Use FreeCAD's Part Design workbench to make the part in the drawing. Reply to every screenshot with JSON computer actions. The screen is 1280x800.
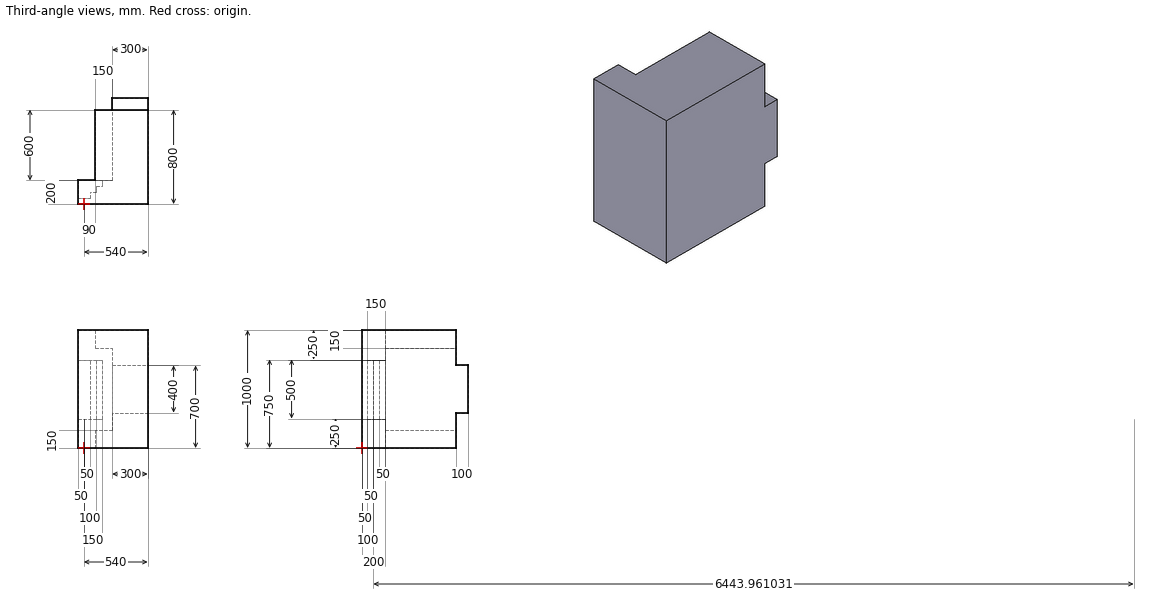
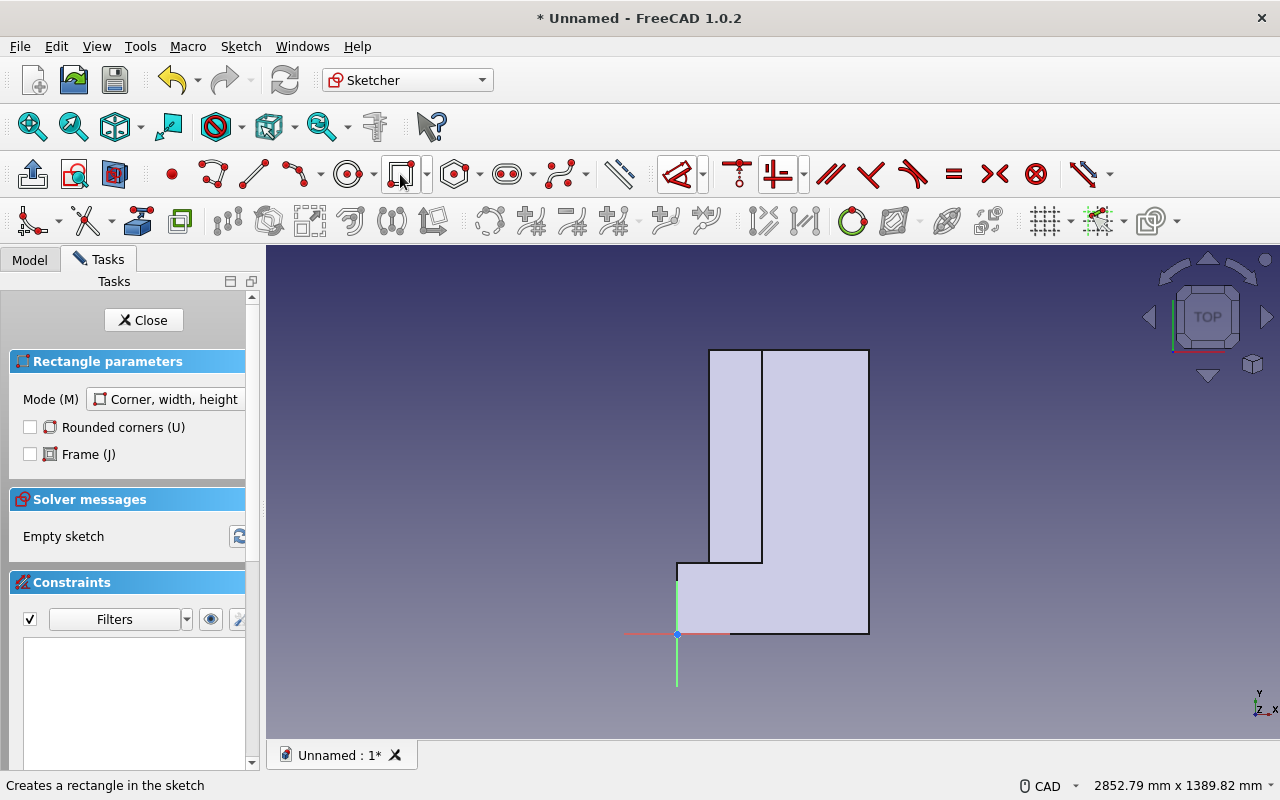
{"action": "left_click", "coordinate": [709, 350]}
{"action": "left_click", "coordinate": [762, 563]}
{"action": "key", "text": "Escape"}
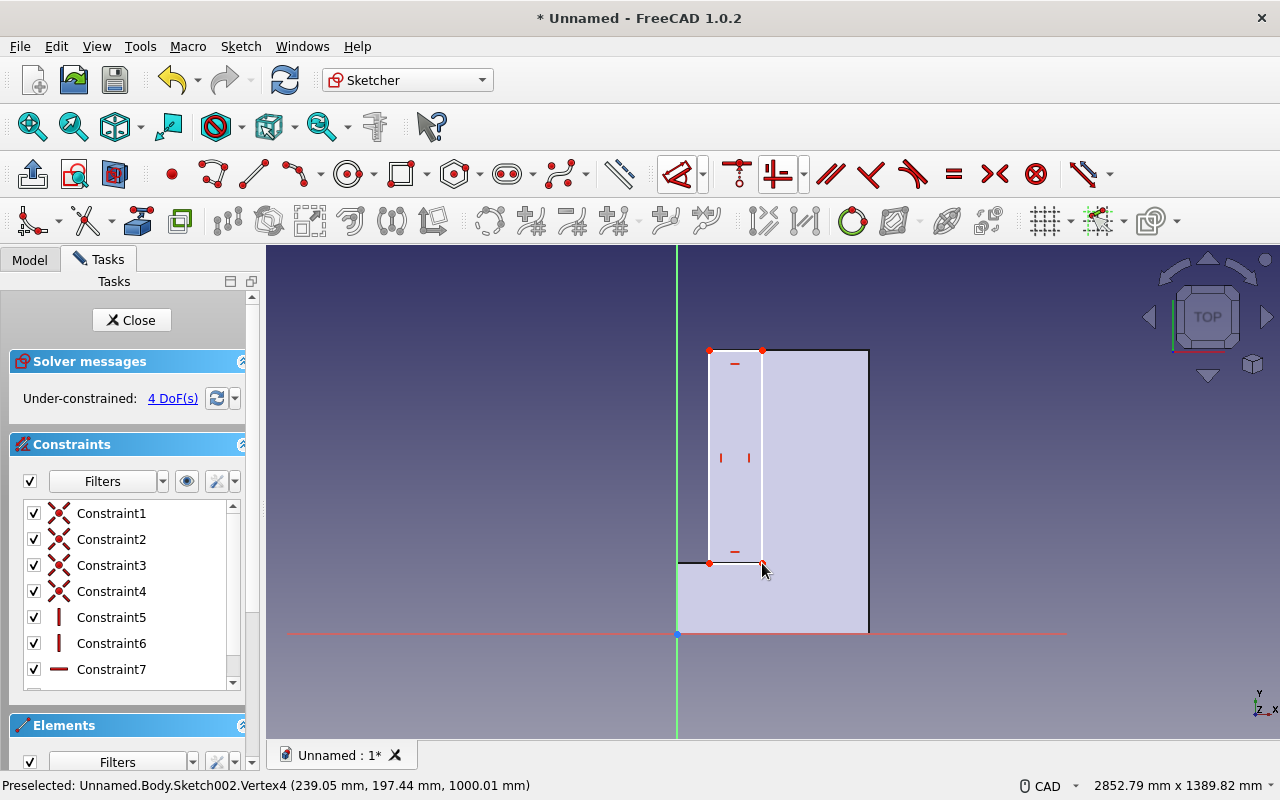
{"action": "left_click", "coordinate": [709, 415]}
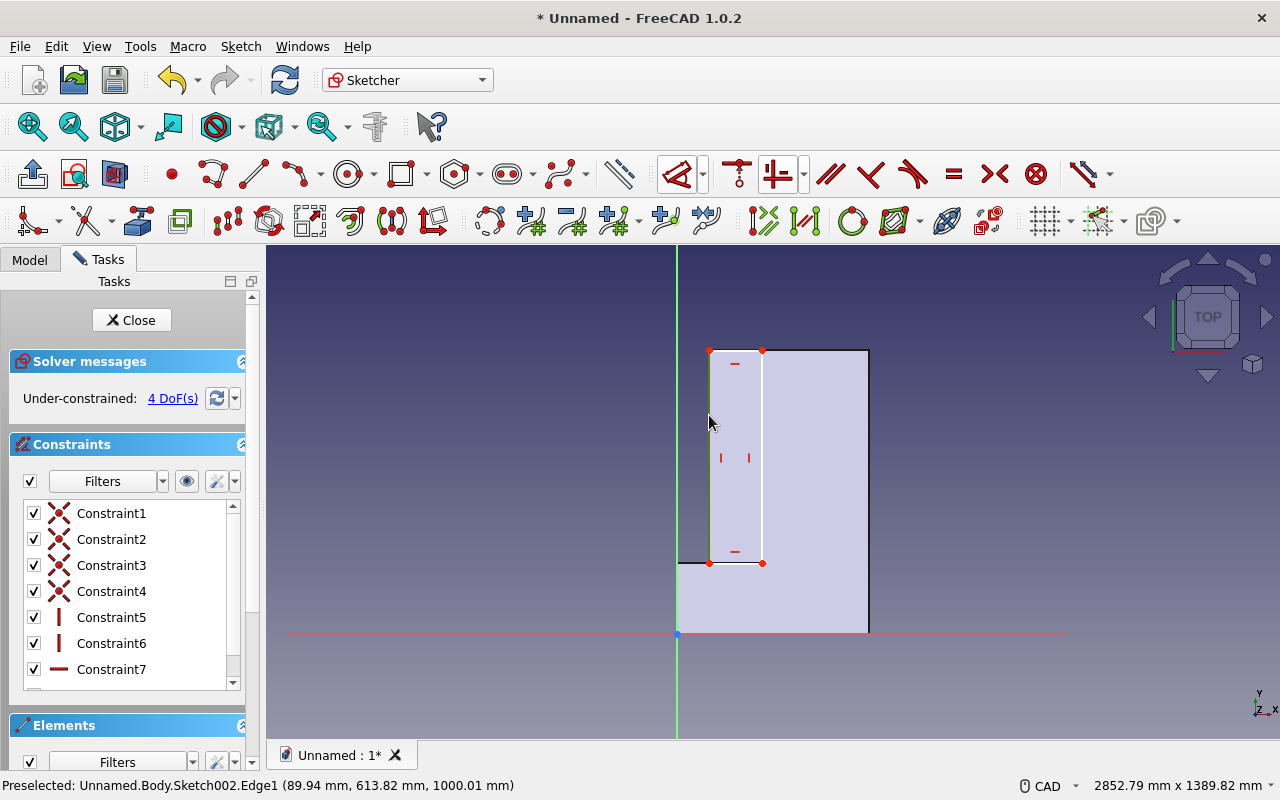
{"action": "key", "text": "i"}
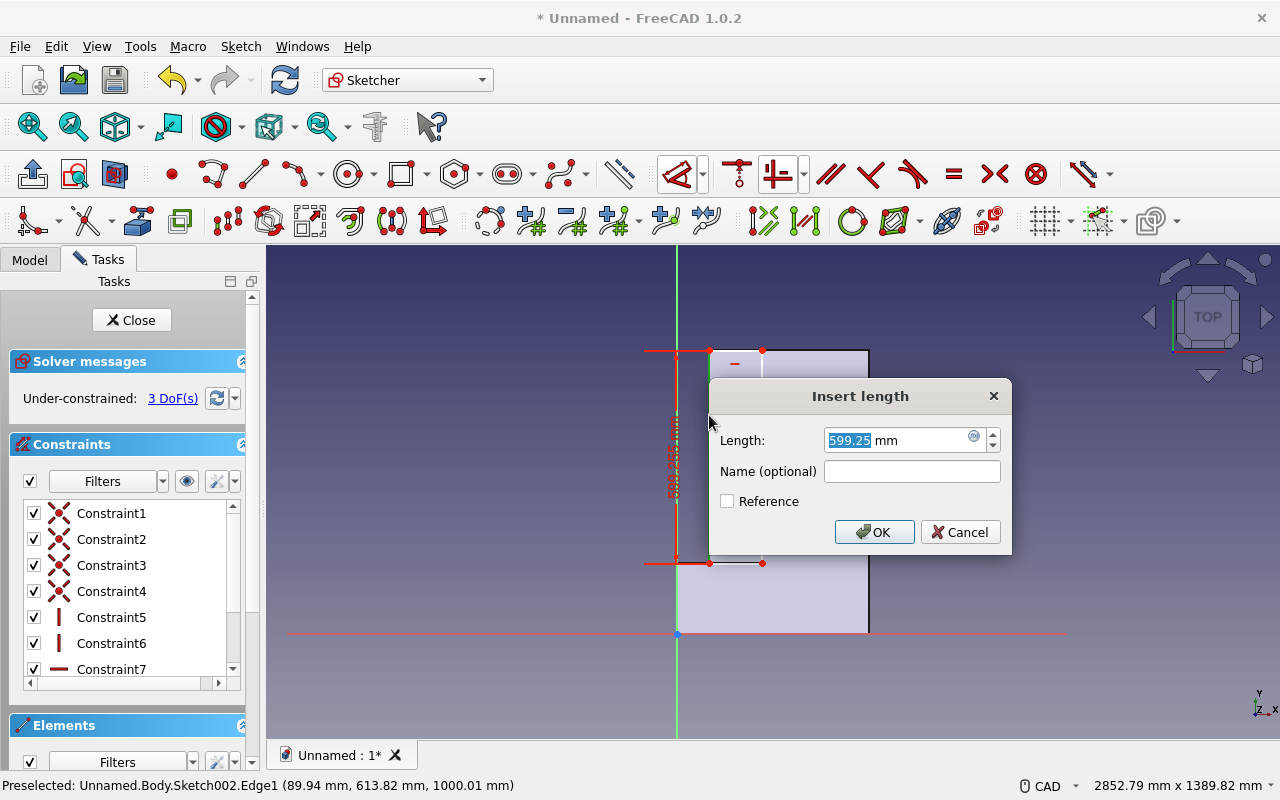
{"action": "type", "text": "600"}
{"action": "key", "text": "Return"}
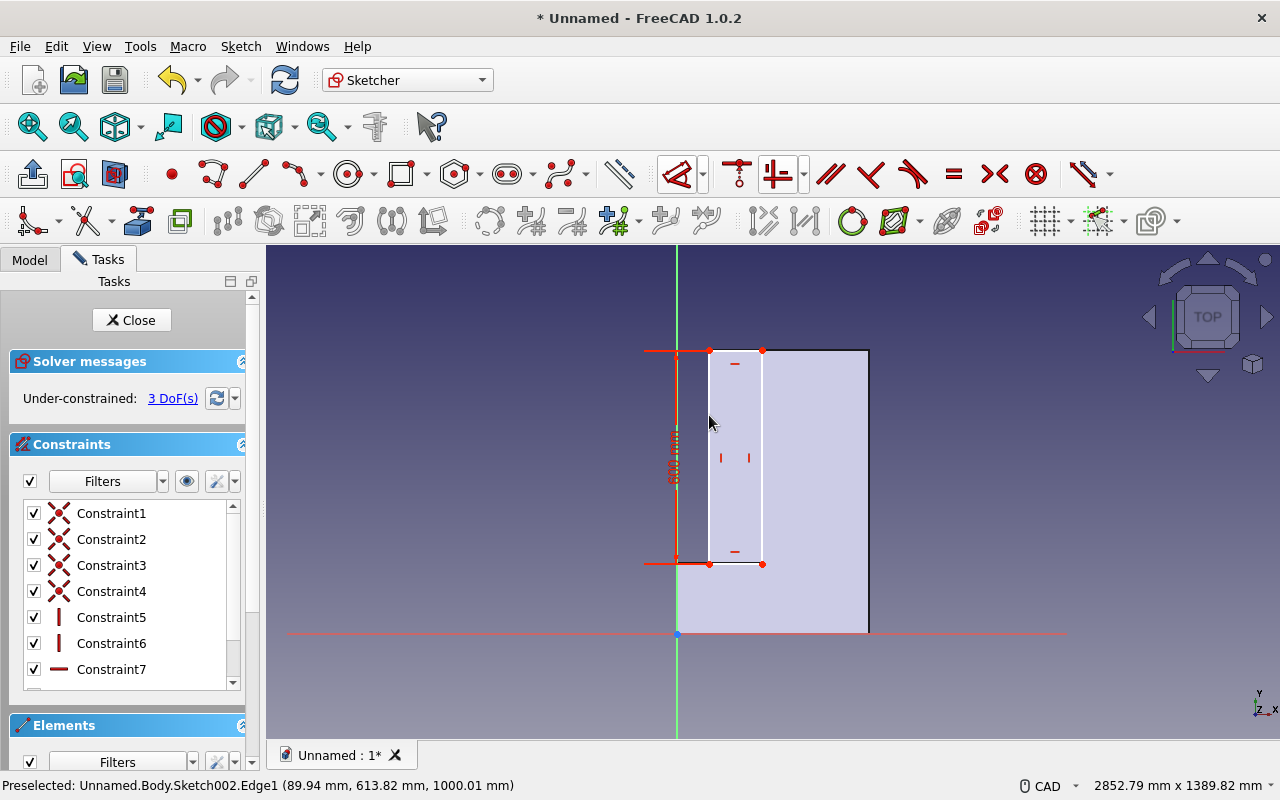
{"action": "left_click", "coordinate": [725, 564]}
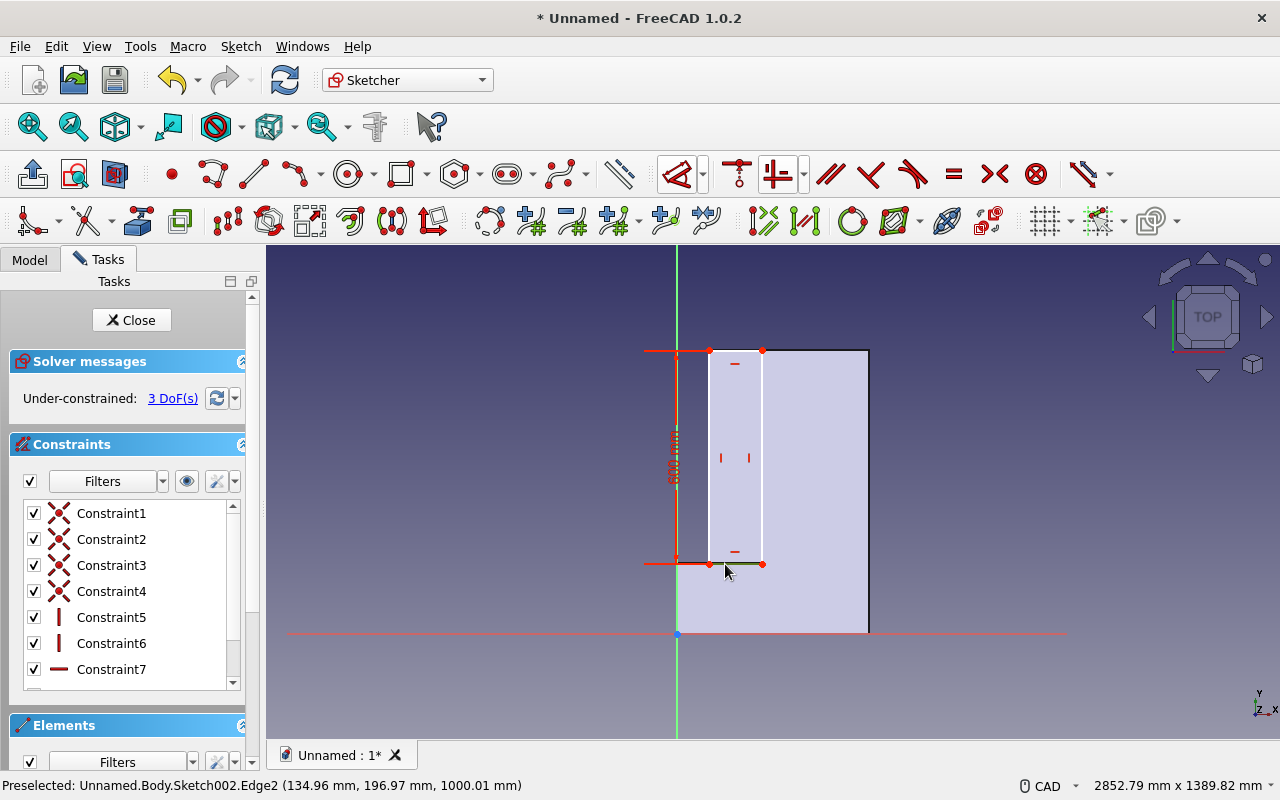
{"action": "key", "text": "l"}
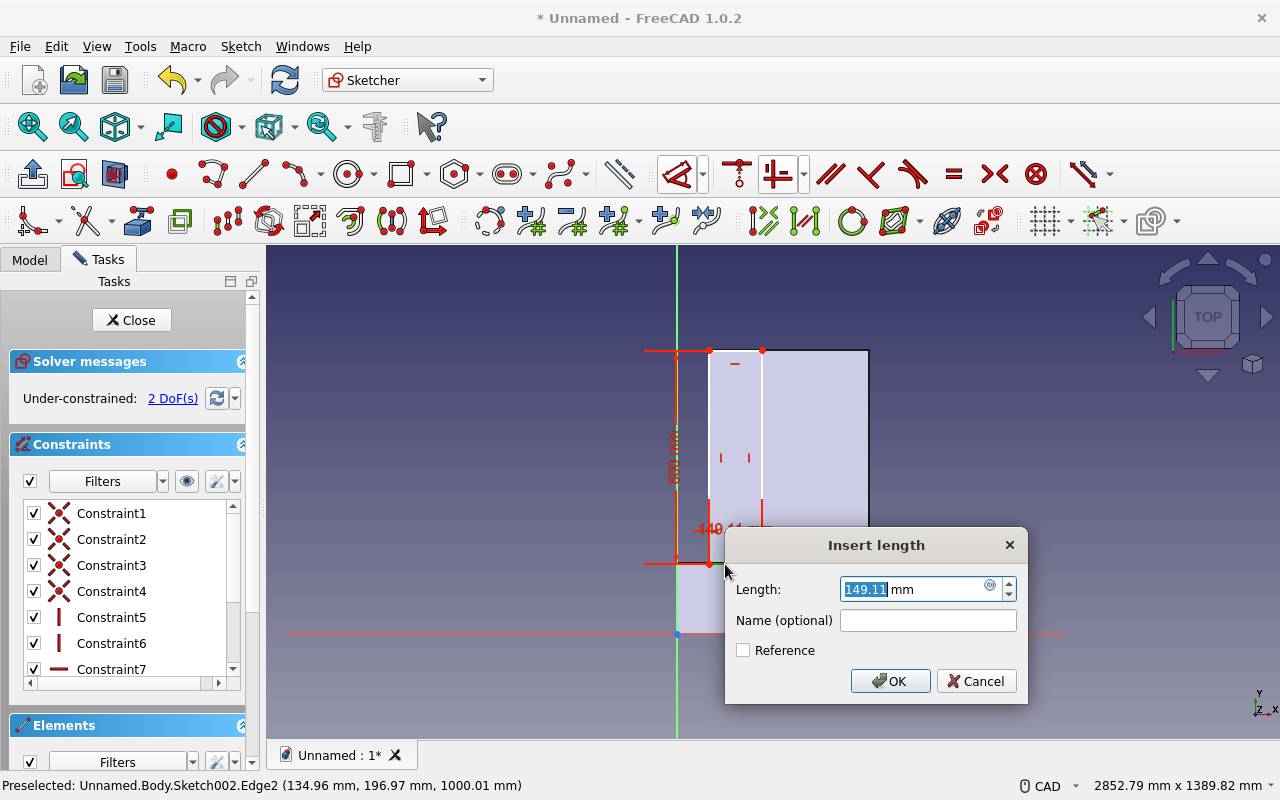
{"action": "type", "text": "150"}
{"action": "key", "text": "Return"}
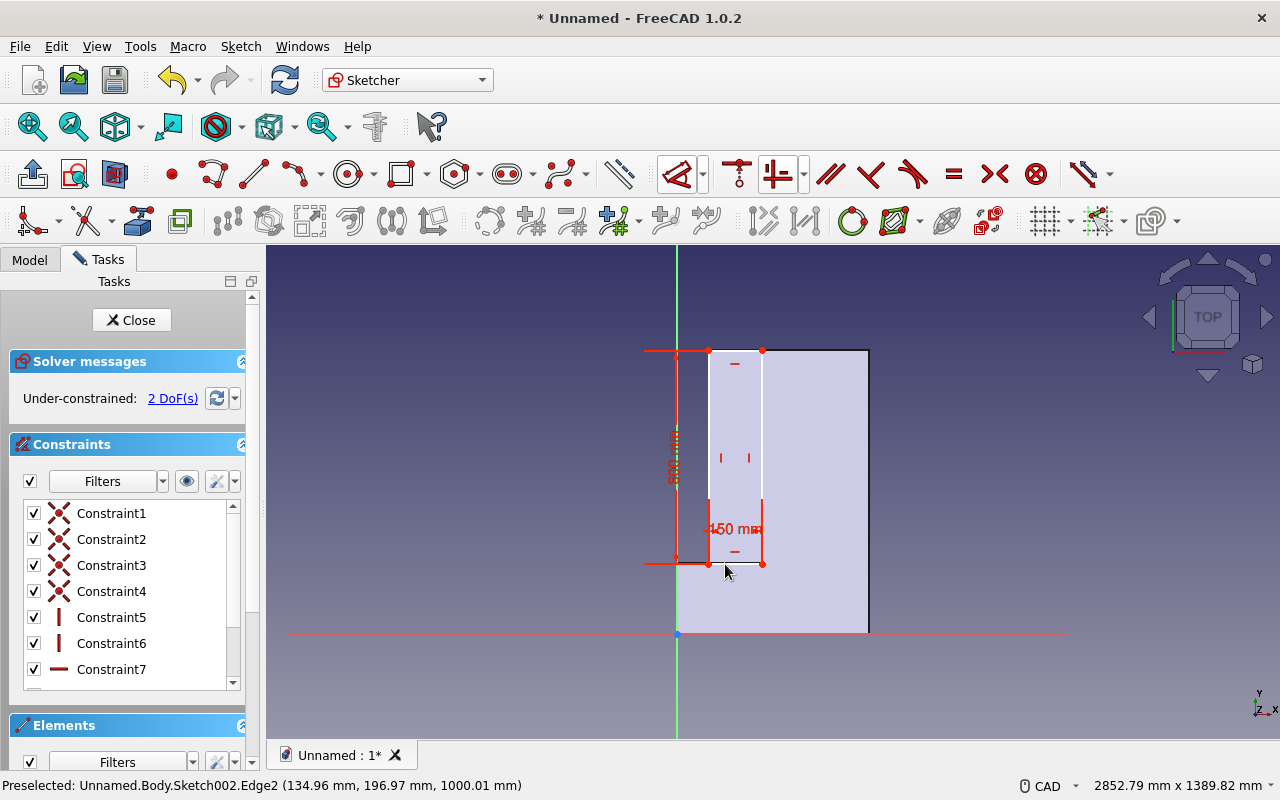
{"action": "scroll", "coordinate": [709, 351], "scroll_direction": "up", "scroll_amount": 2}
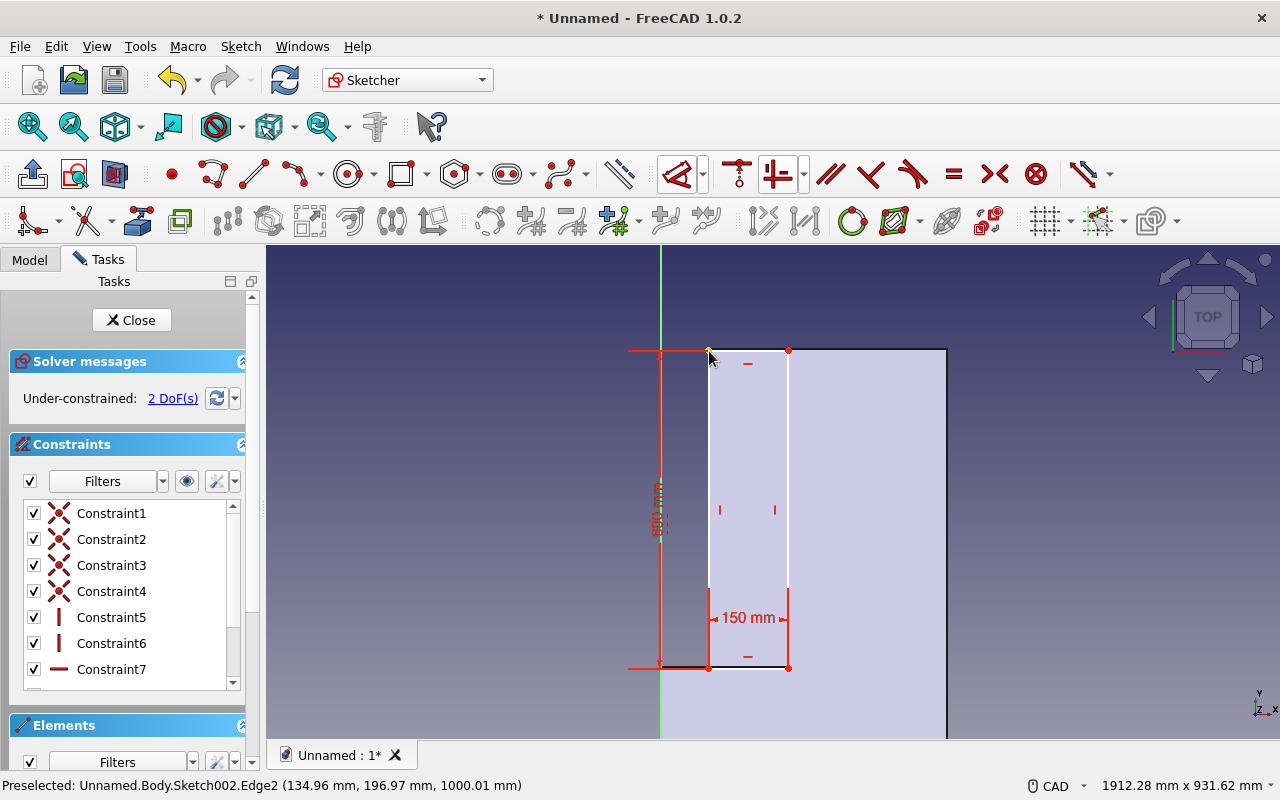
{"action": "left_click", "coordinate": [709, 351]}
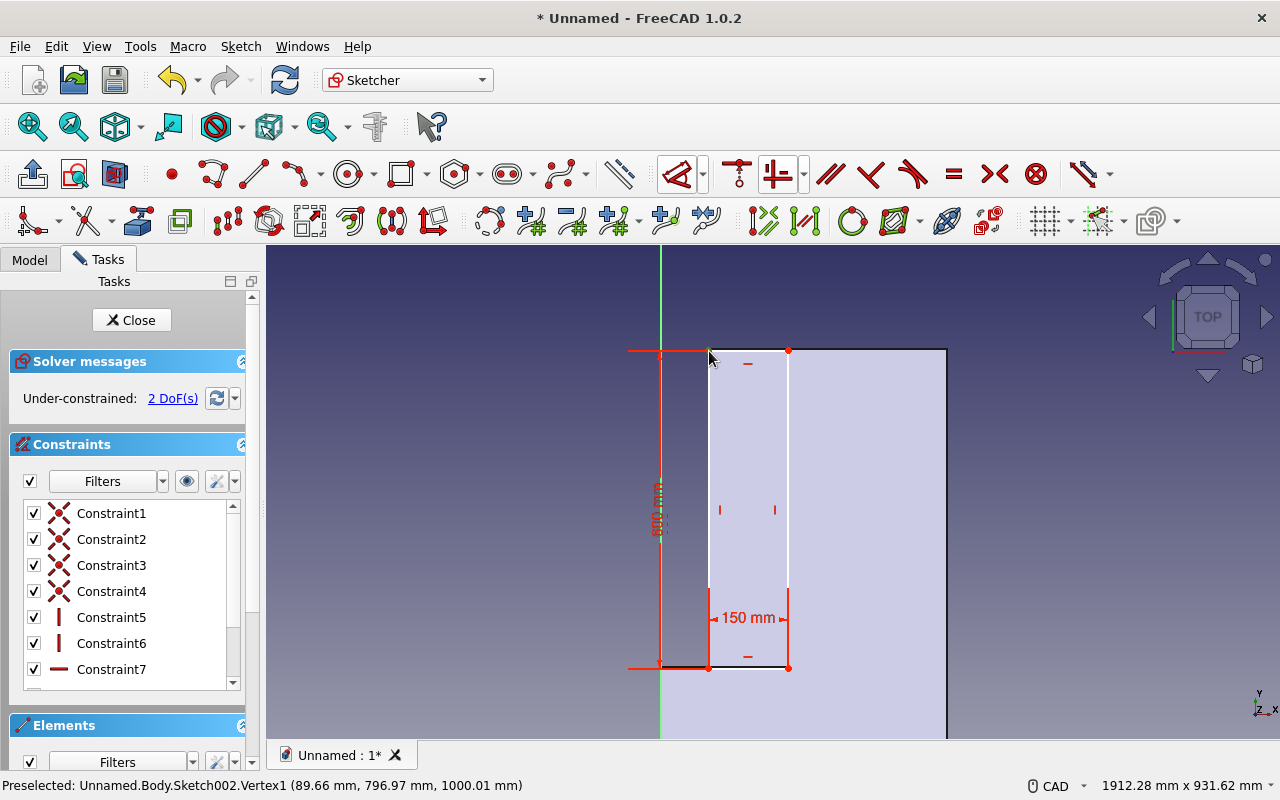
{"action": "key", "text": "l"}